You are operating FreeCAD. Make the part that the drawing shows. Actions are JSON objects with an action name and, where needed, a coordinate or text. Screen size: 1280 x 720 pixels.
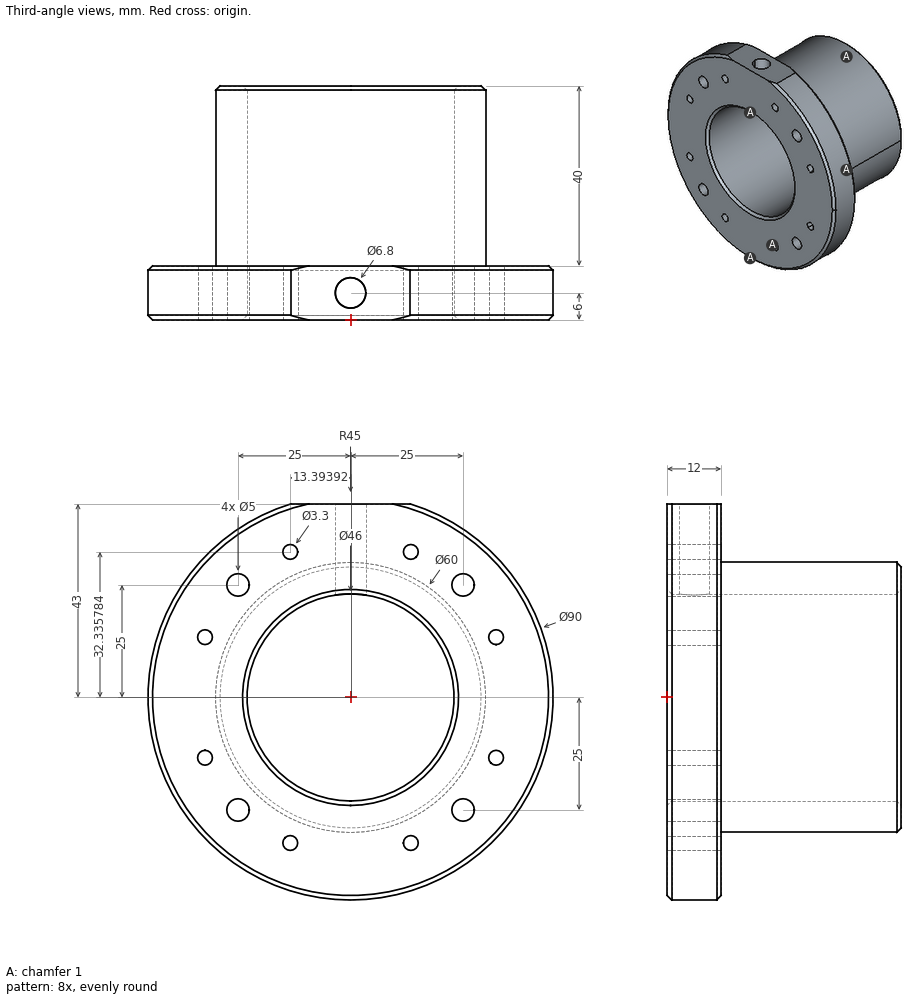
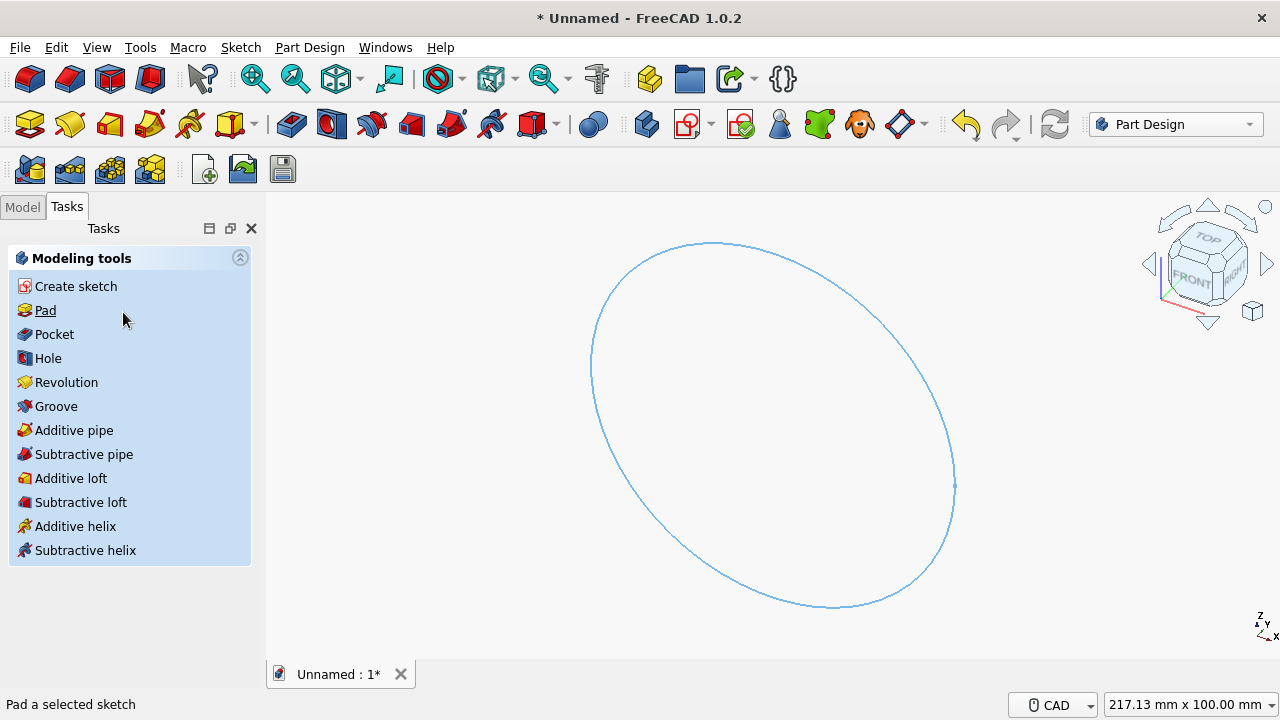
{"action": "left_click", "coordinate": [30, 124]}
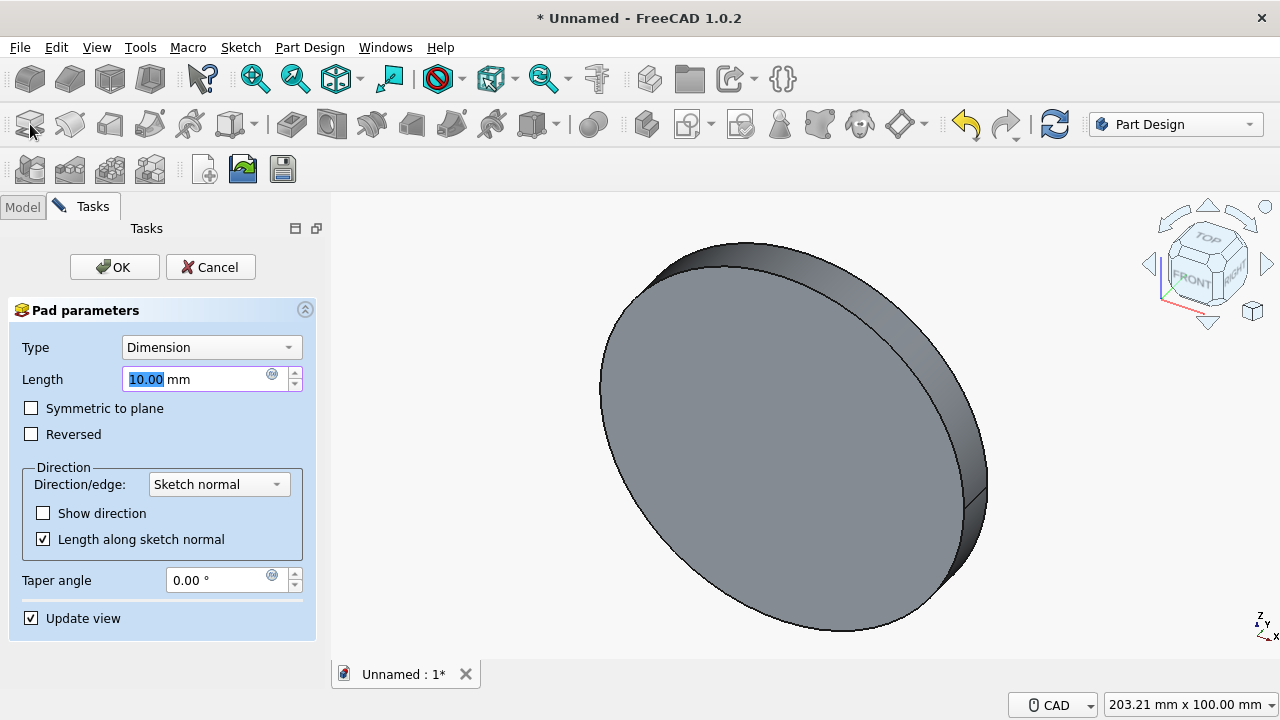
{"action": "type", "text": "12"}
{"action": "key", "text": "Tab"}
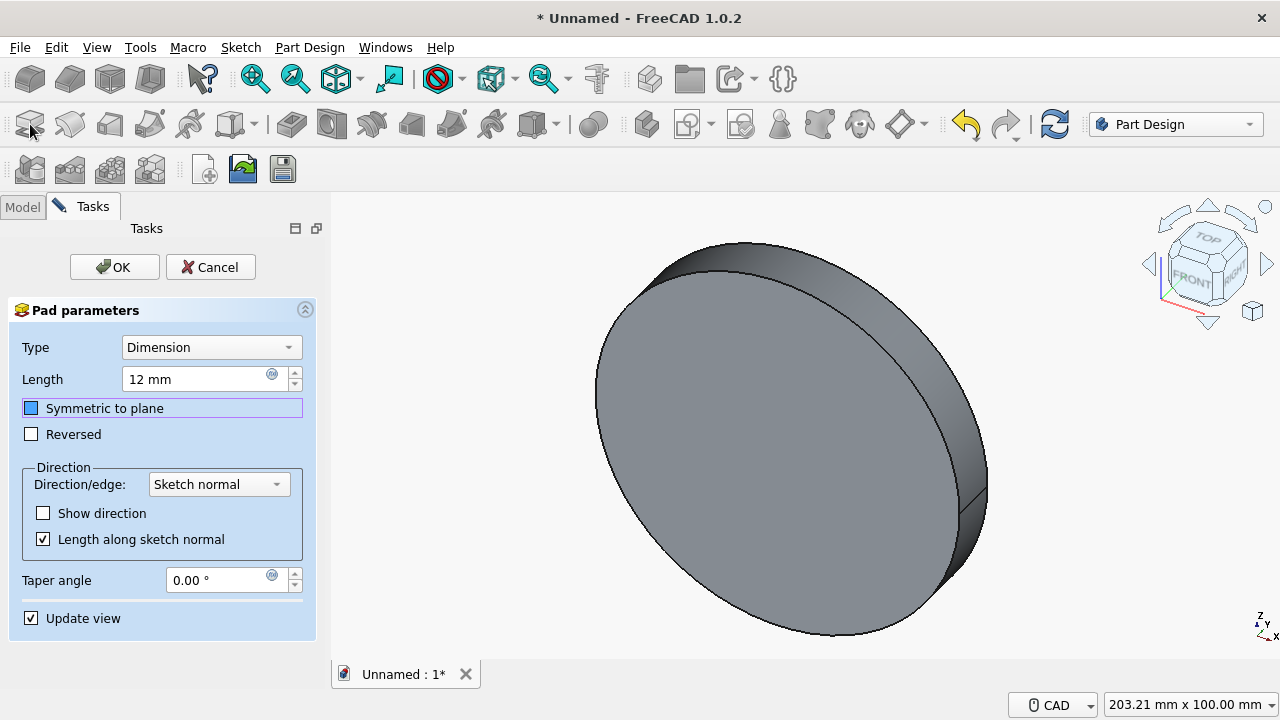
{"action": "left_click", "coordinate": [30, 434]}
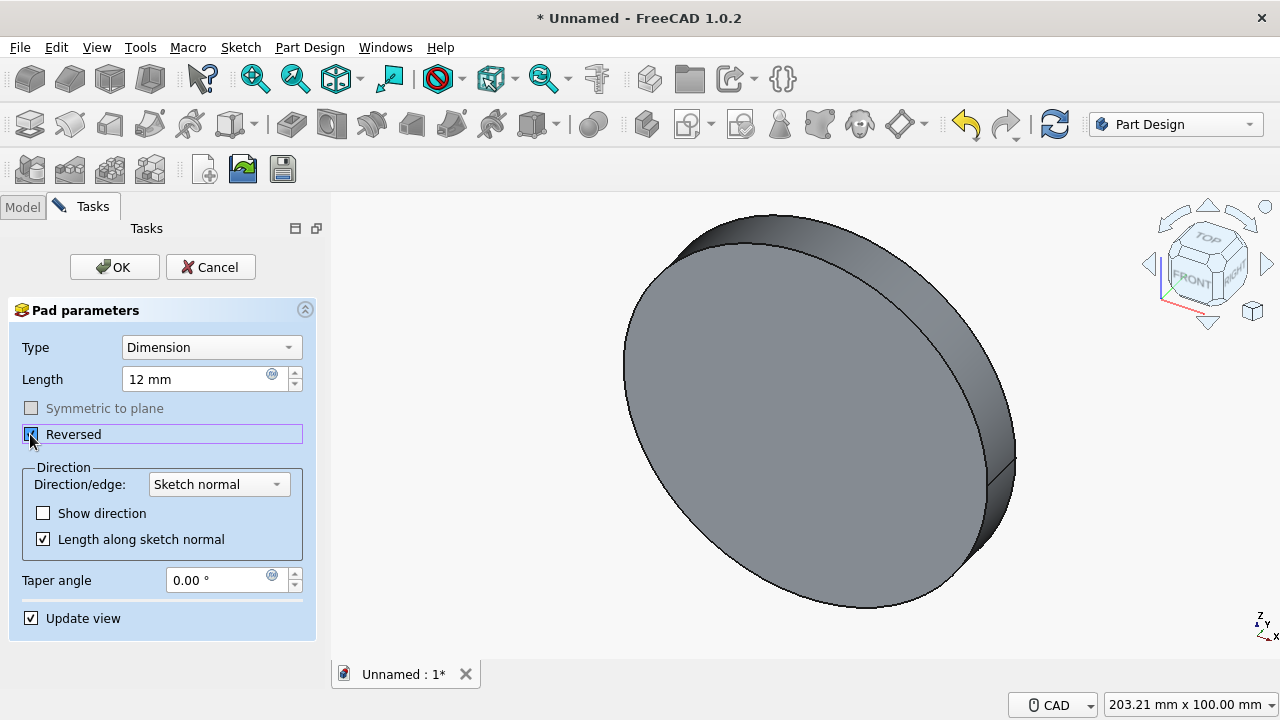
{"action": "left_click", "coordinate": [115, 267]}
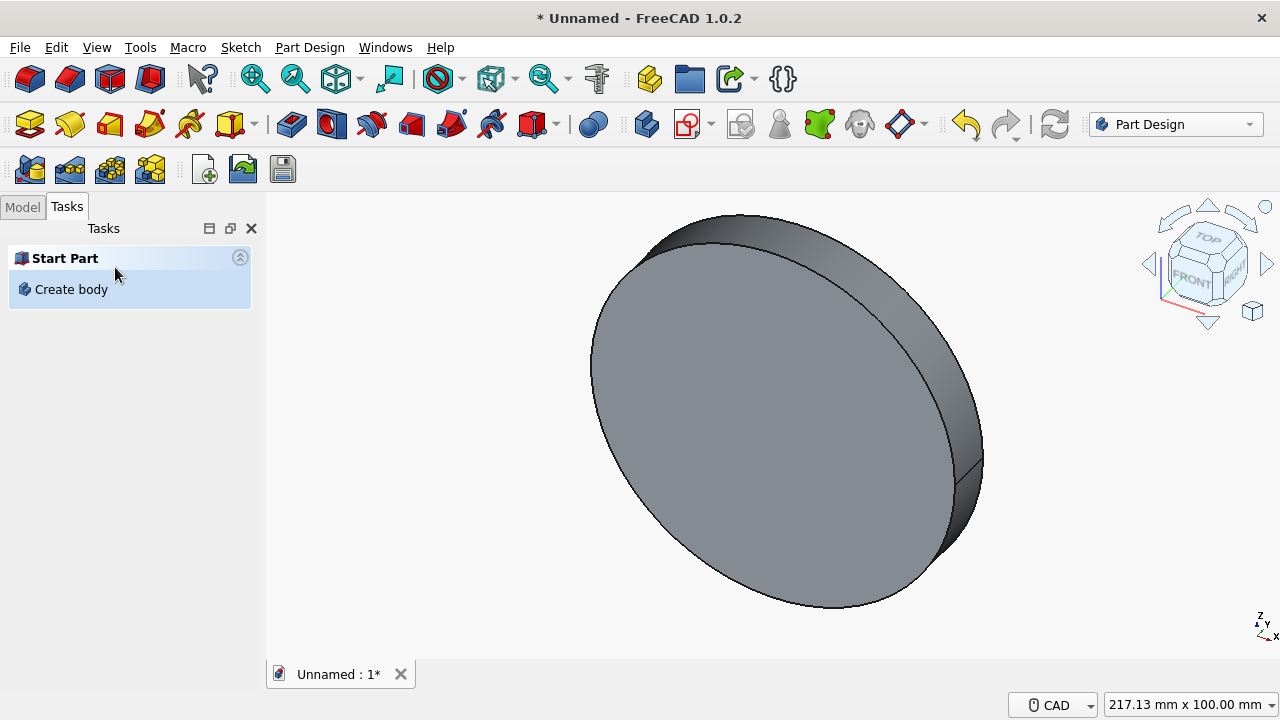
{"action": "key", "text": "v f"}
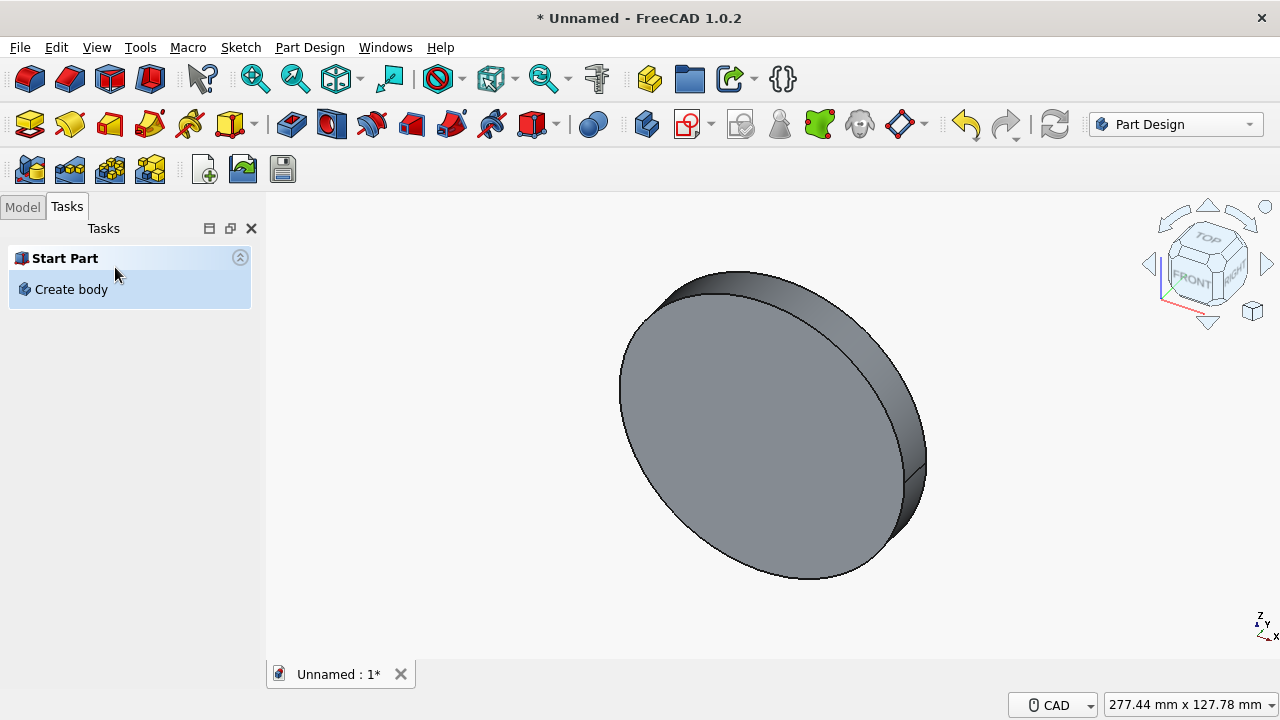
{"action": "key", "text": "4"}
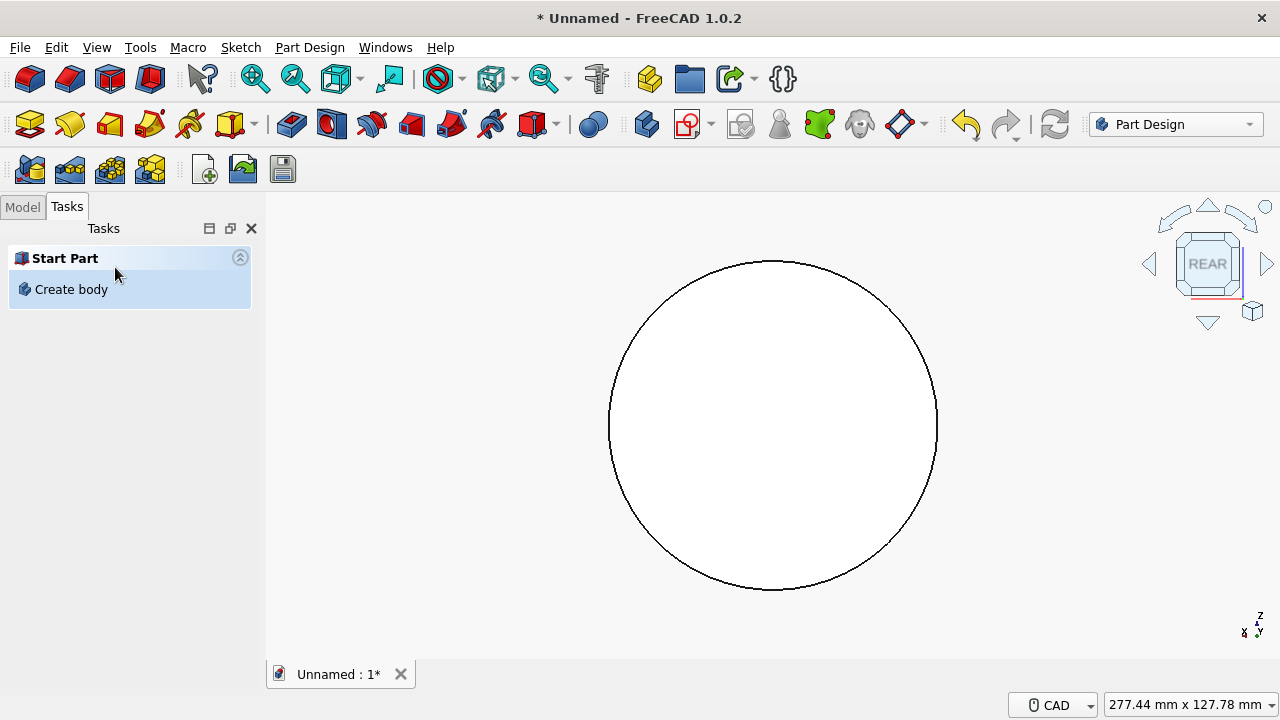
{"action": "left_click", "coordinate": [773, 424]}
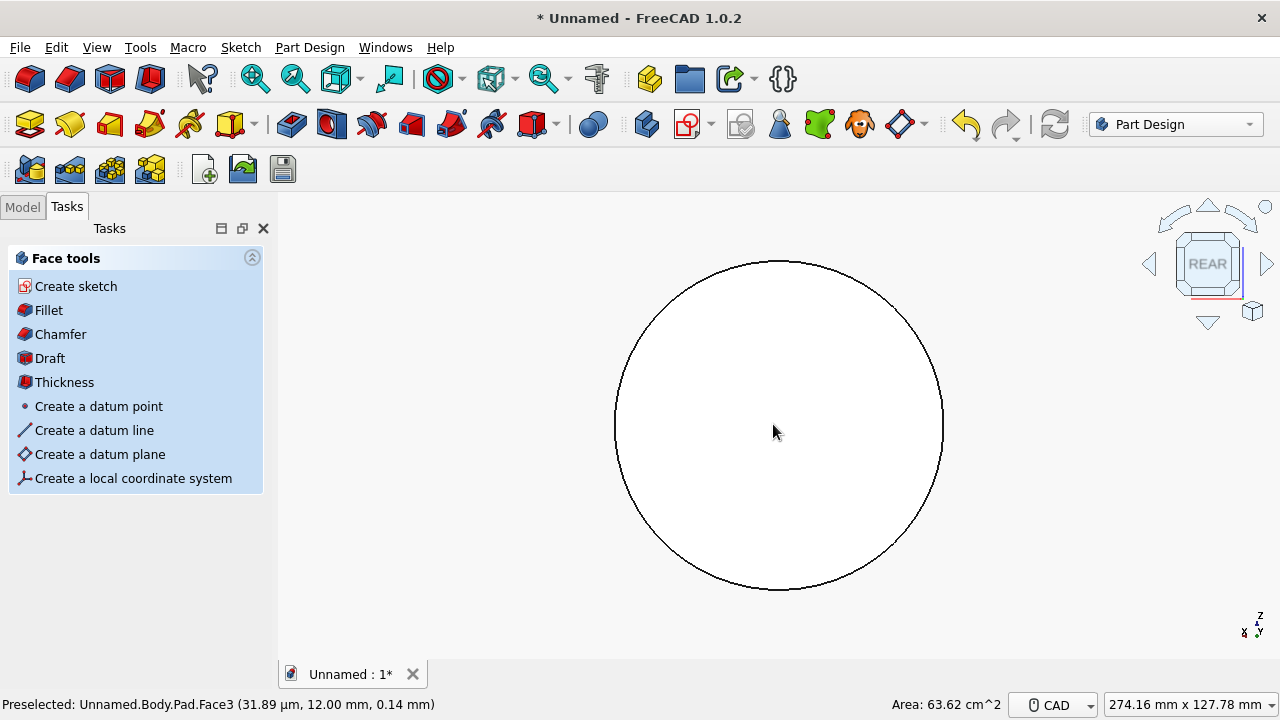
{"action": "left_click", "coordinate": [688, 124]}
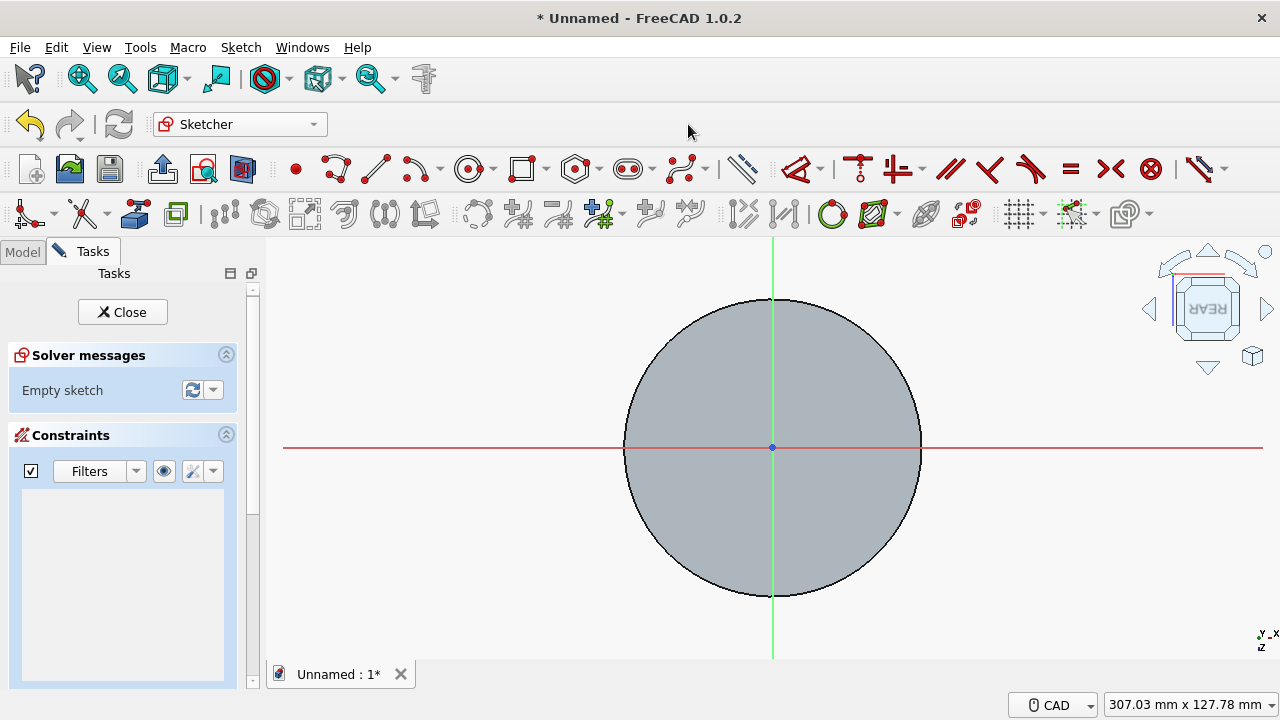
{"action": "left_click", "coordinate": [470, 170]}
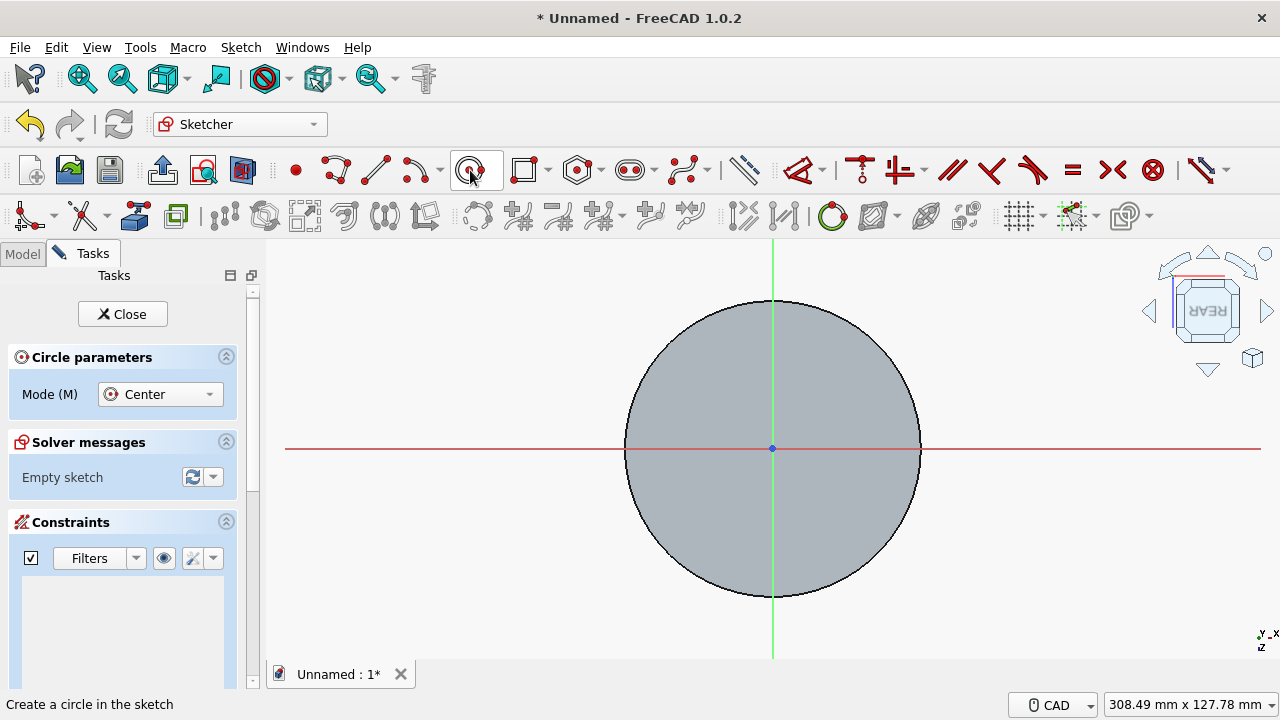
{"action": "left_click", "coordinate": [773, 449]}
{"action": "left_click", "coordinate": [843, 379]}
{"action": "key", "text": "Escape"}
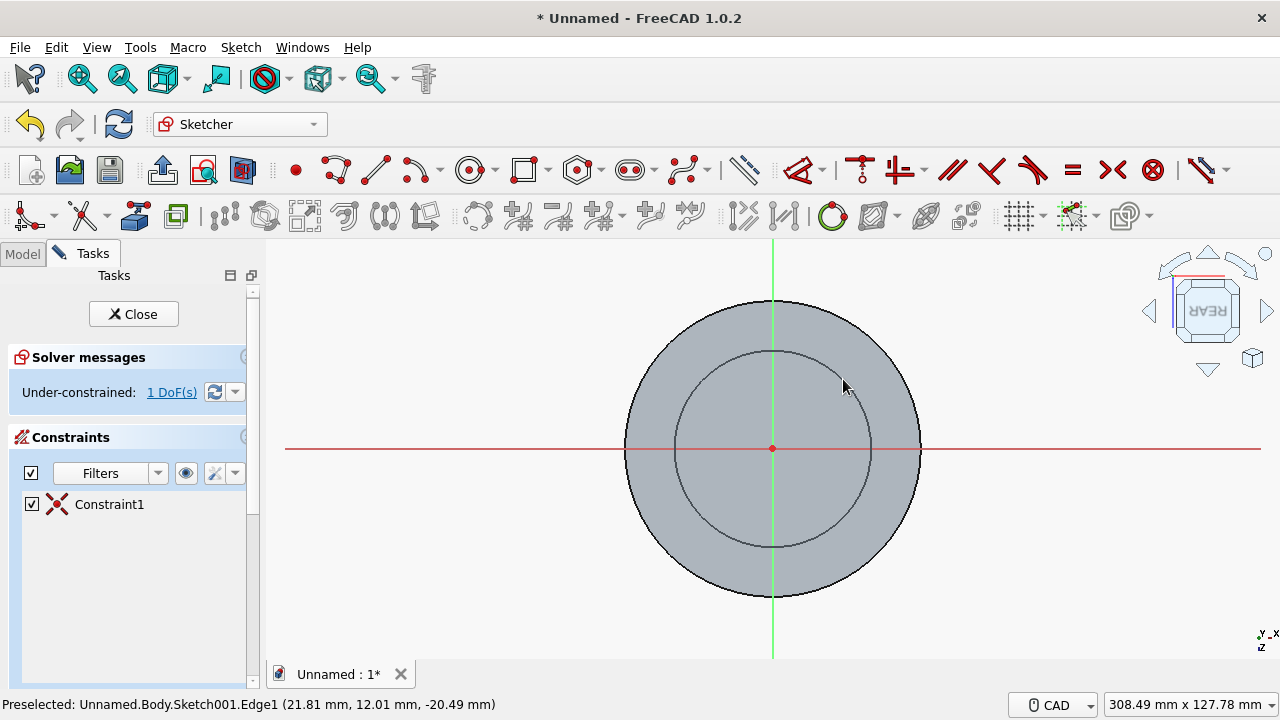
{"action": "left_click", "coordinate": [798, 170]}